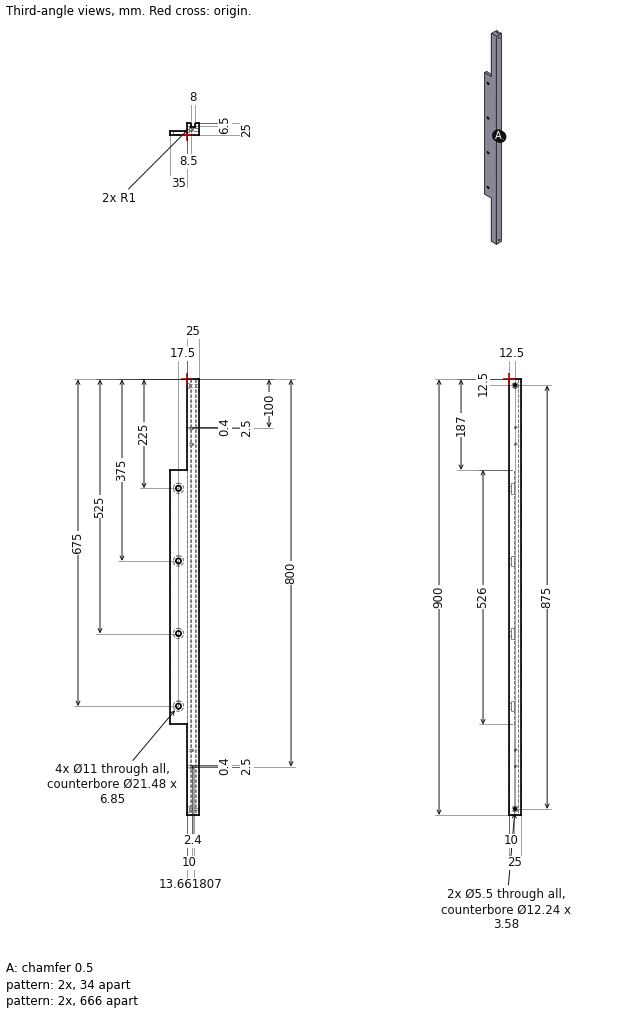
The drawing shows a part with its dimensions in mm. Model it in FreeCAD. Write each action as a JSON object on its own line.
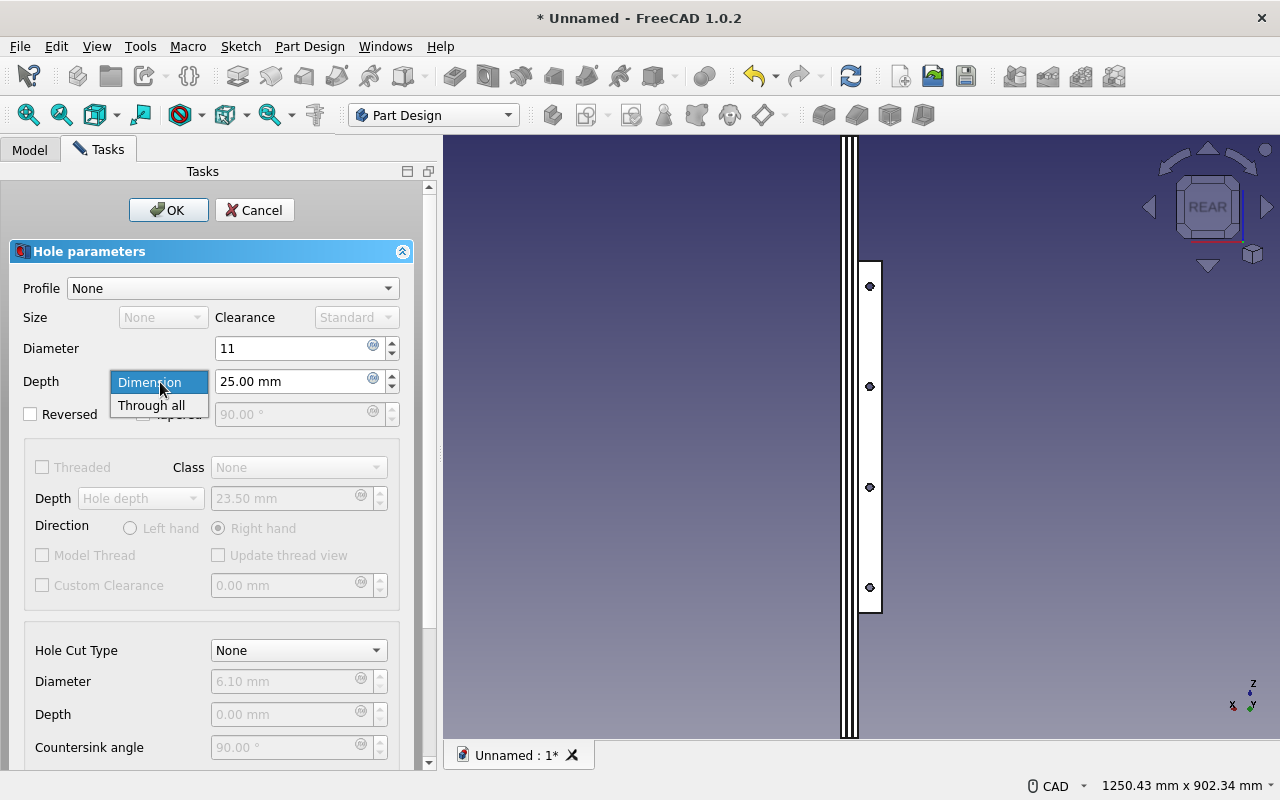
{"action": "left_click", "coordinate": [158, 406]}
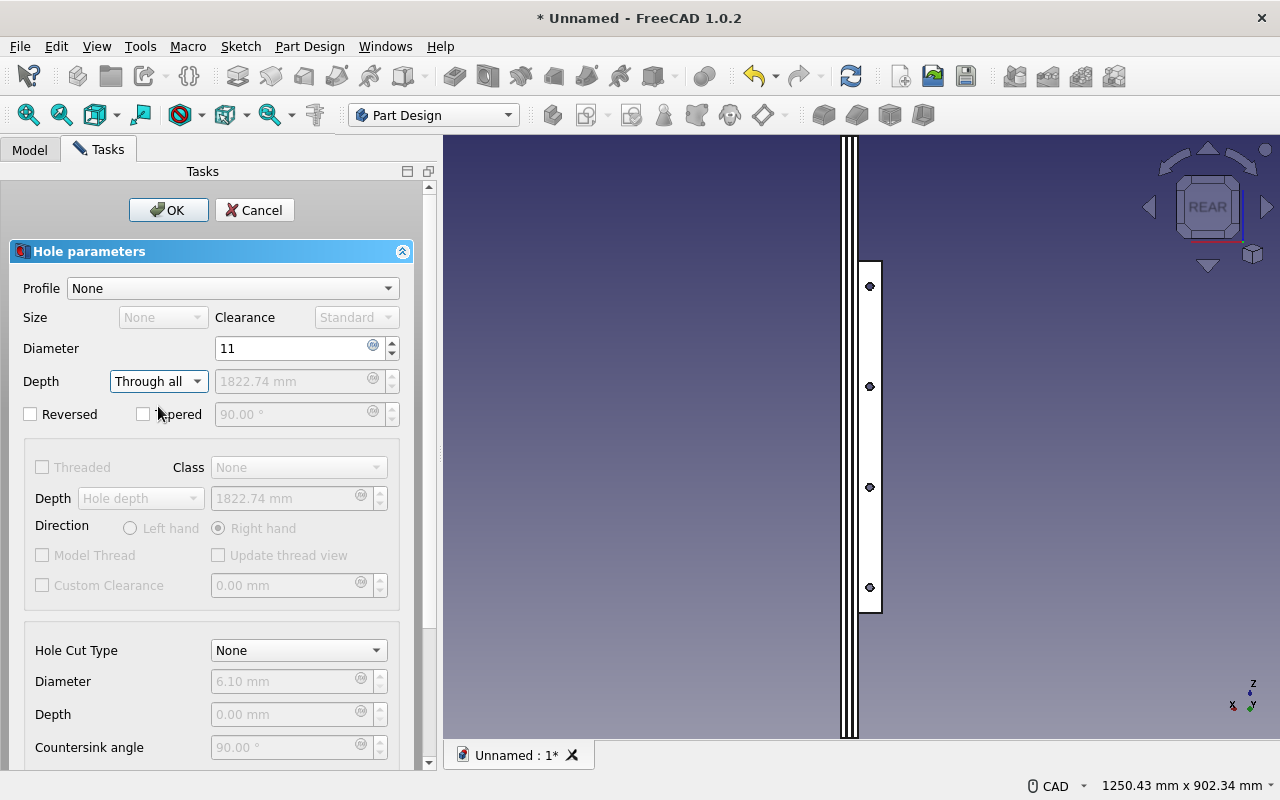
{"action": "left_click", "coordinate": [300, 650]}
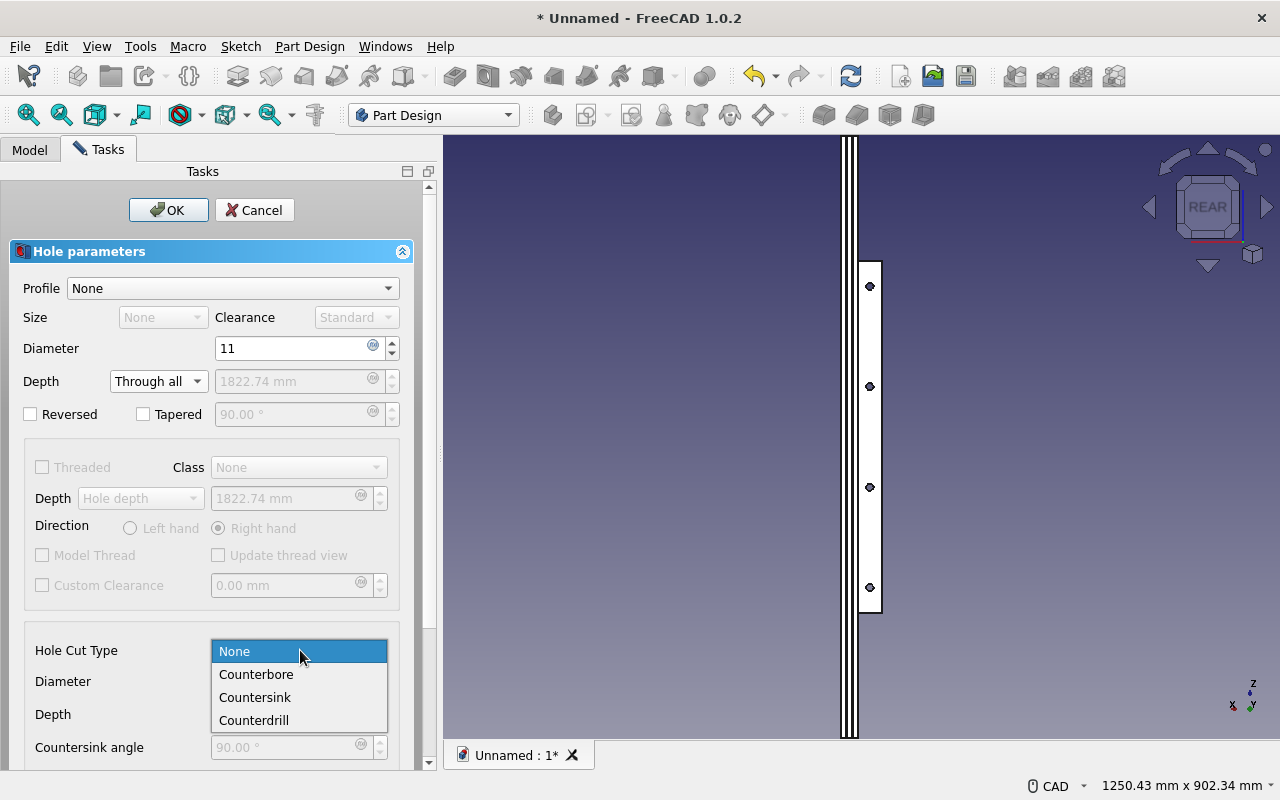
{"action": "left_click", "coordinate": [298, 674]}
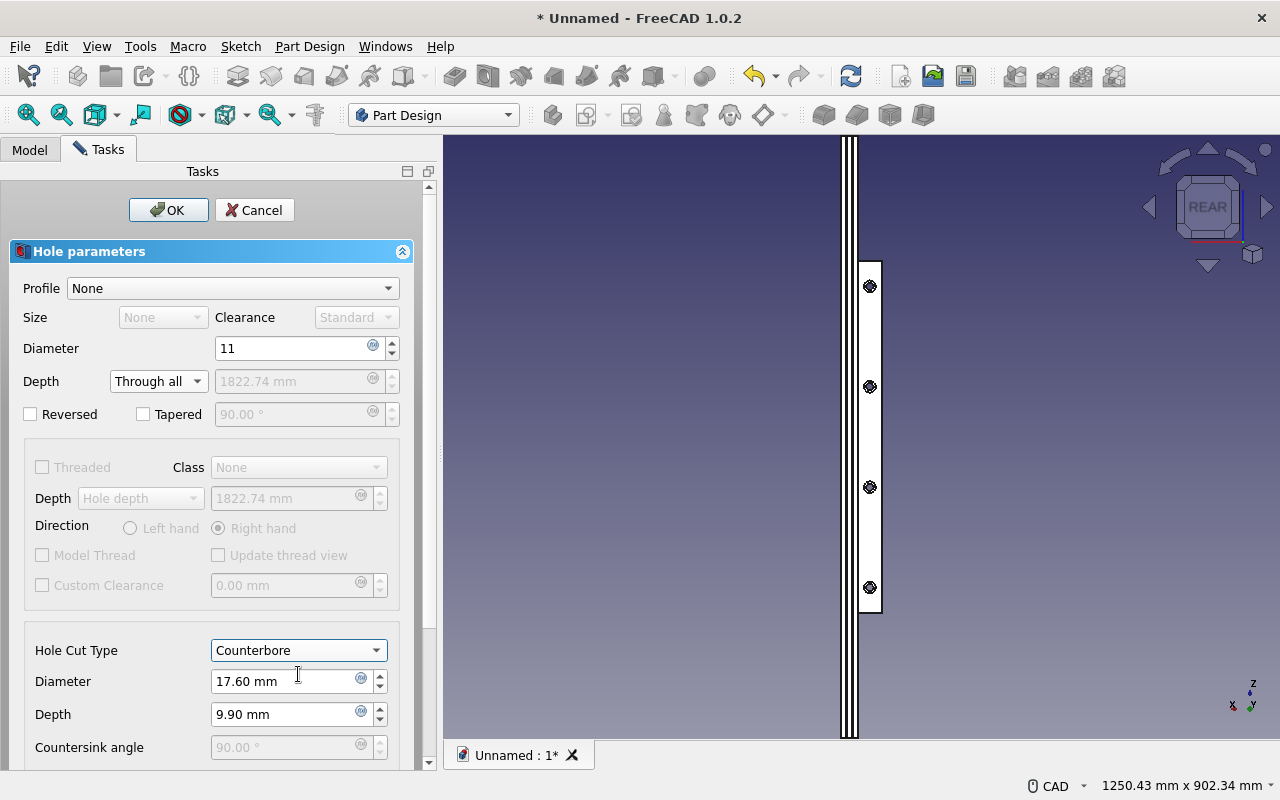
{"action": "triple_click", "coordinate": [292, 682]}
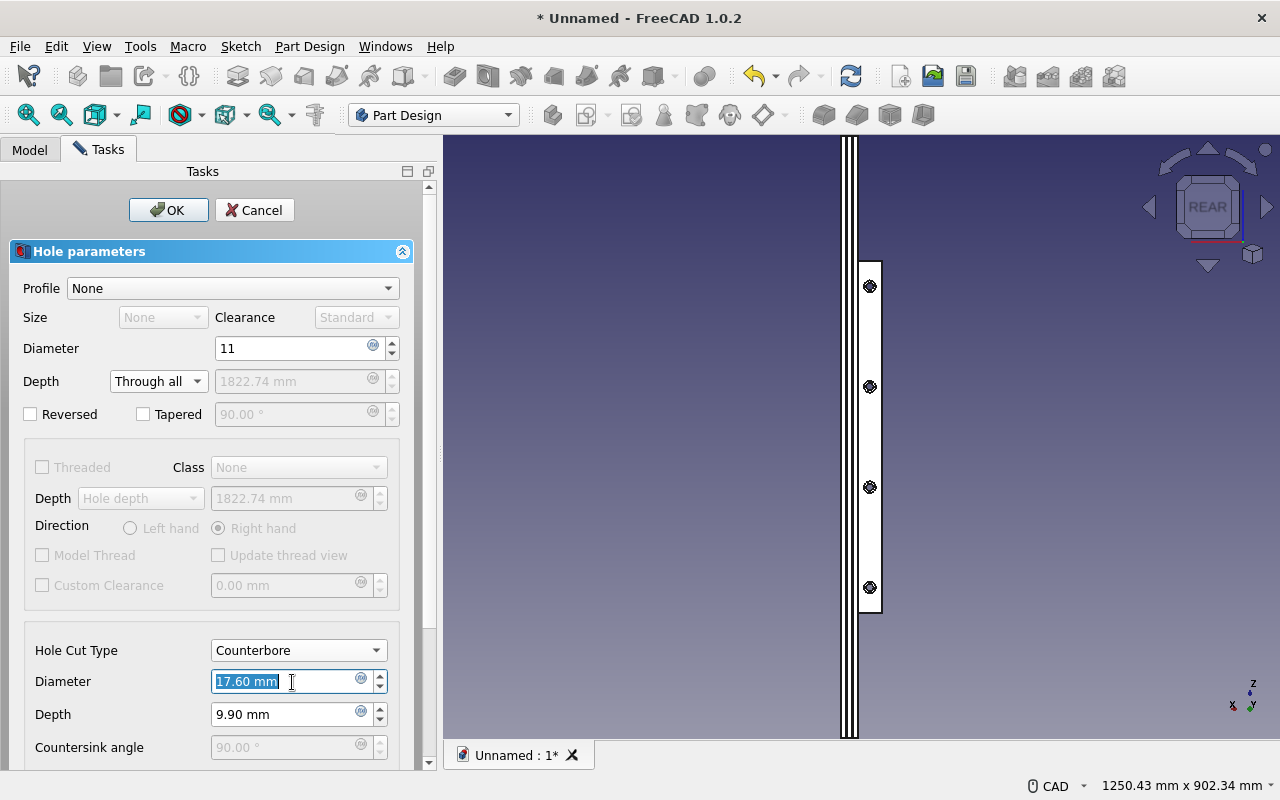
{"action": "type", "text": "21.48"}
{"action": "key", "text": "Tab"}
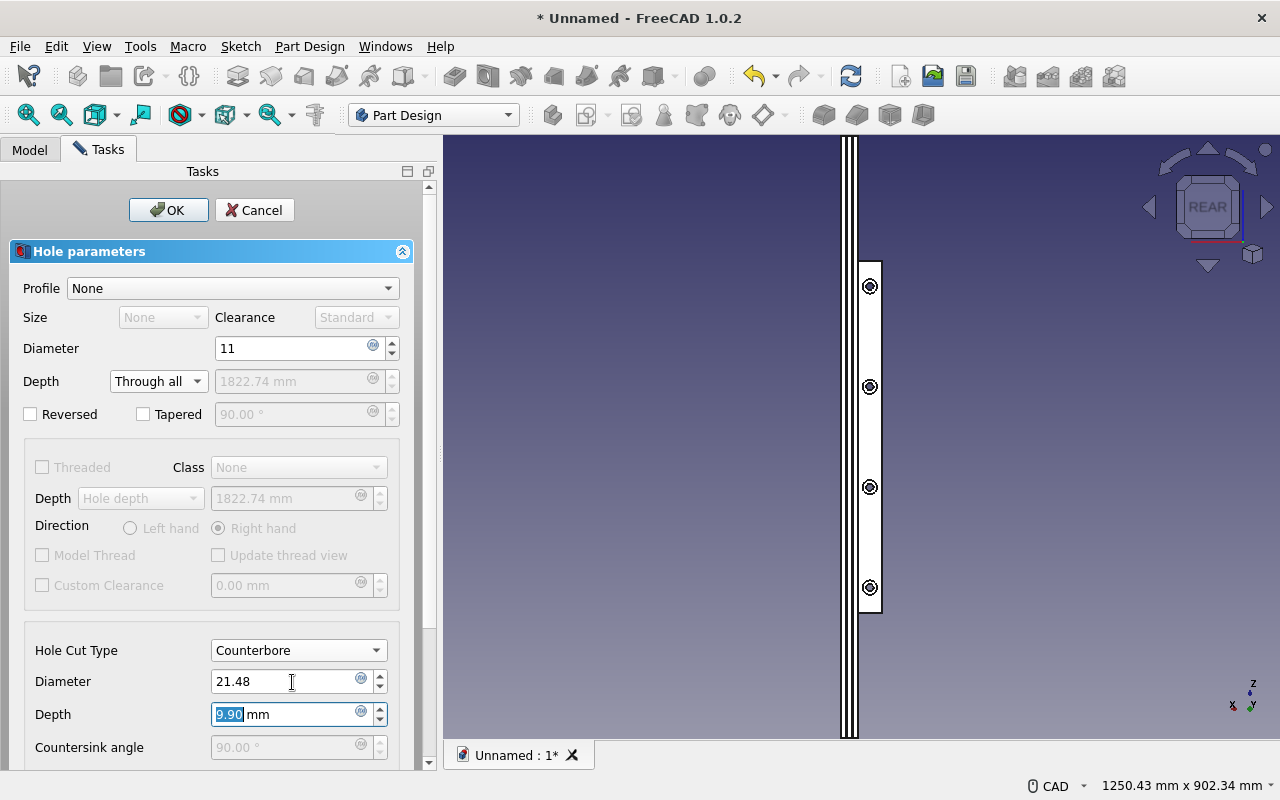
{"action": "type", "text": "6.85"}
{"action": "key", "text": "Tab"}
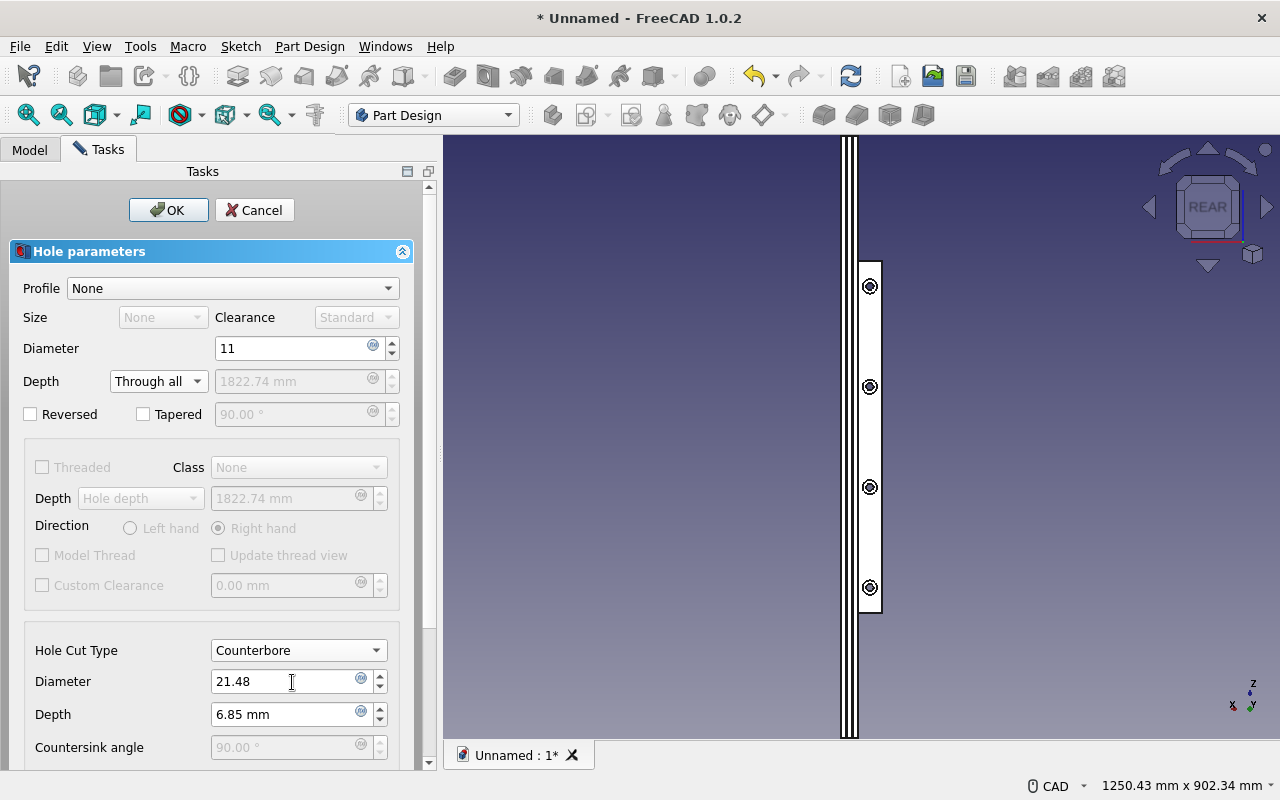
{"action": "left_click", "coordinate": [169, 210]}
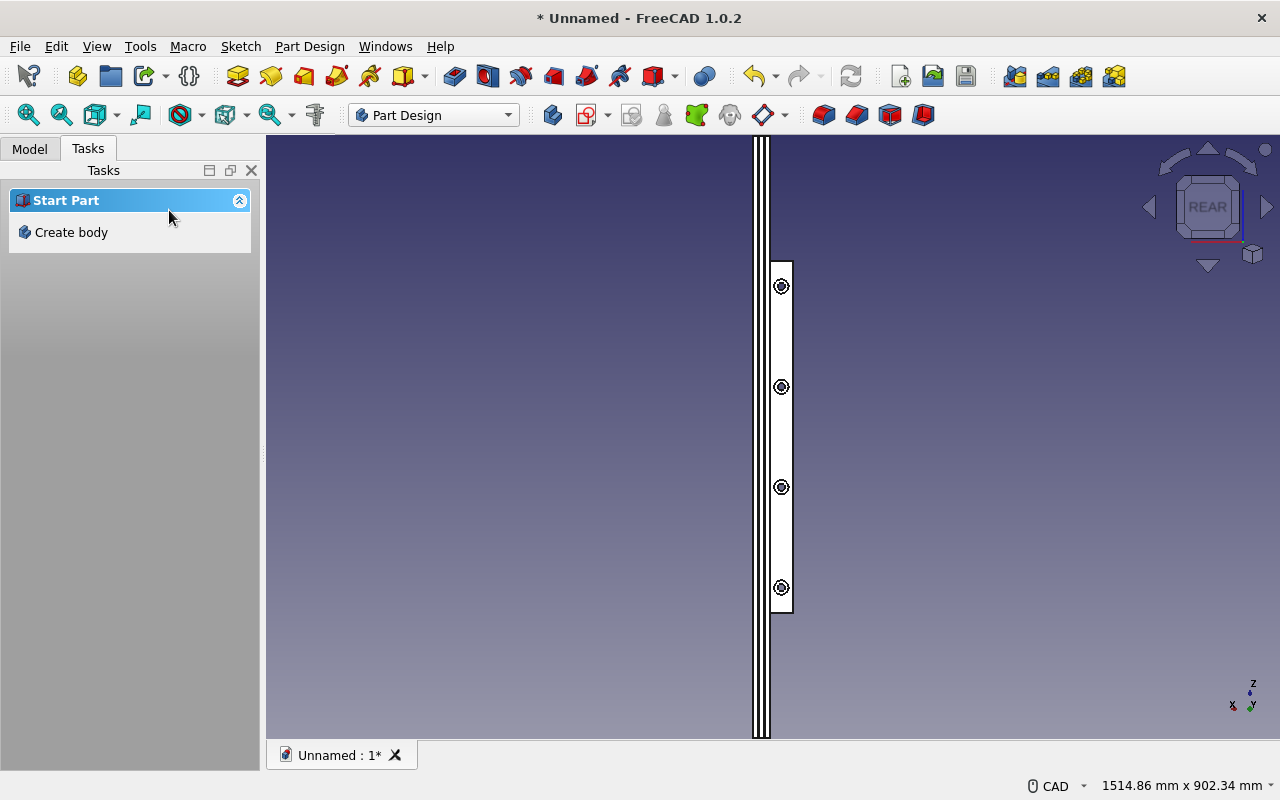
{"action": "key", "text": "6"}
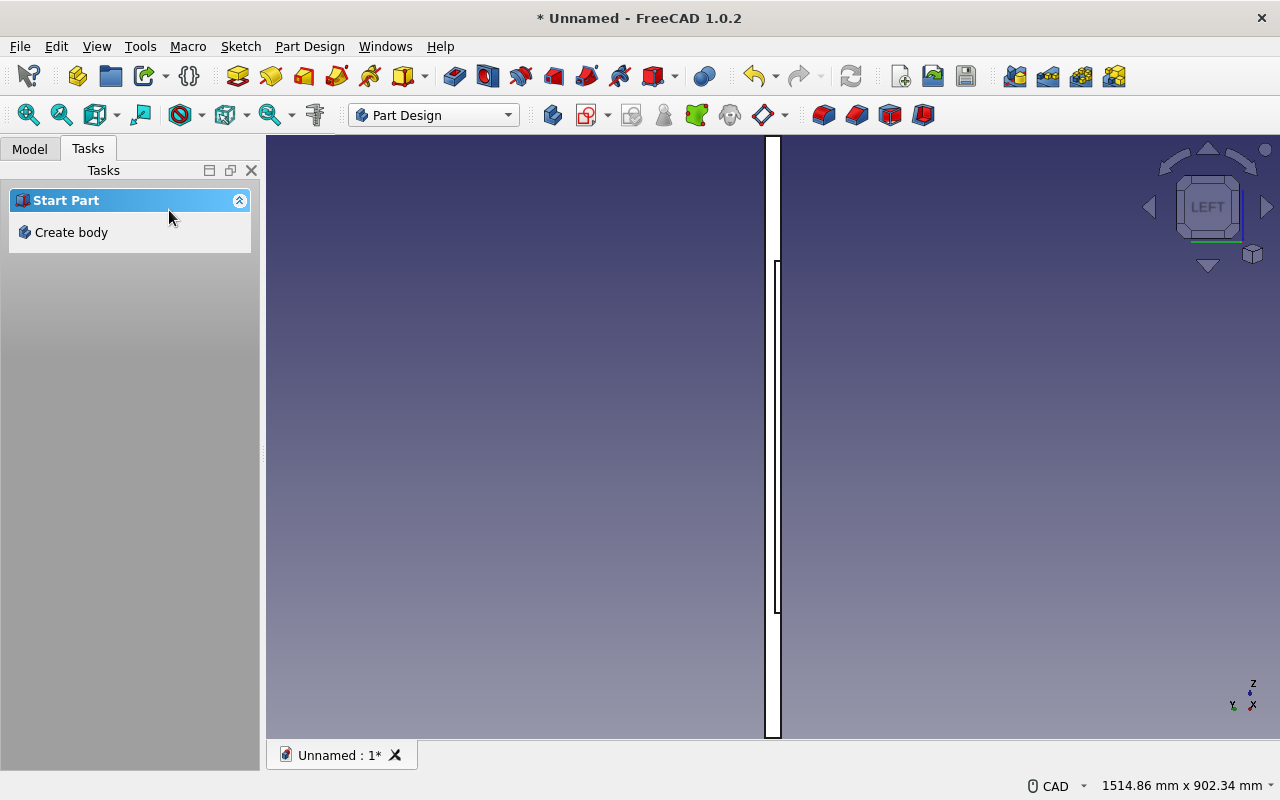
{"action": "left_click", "coordinate": [773, 694]}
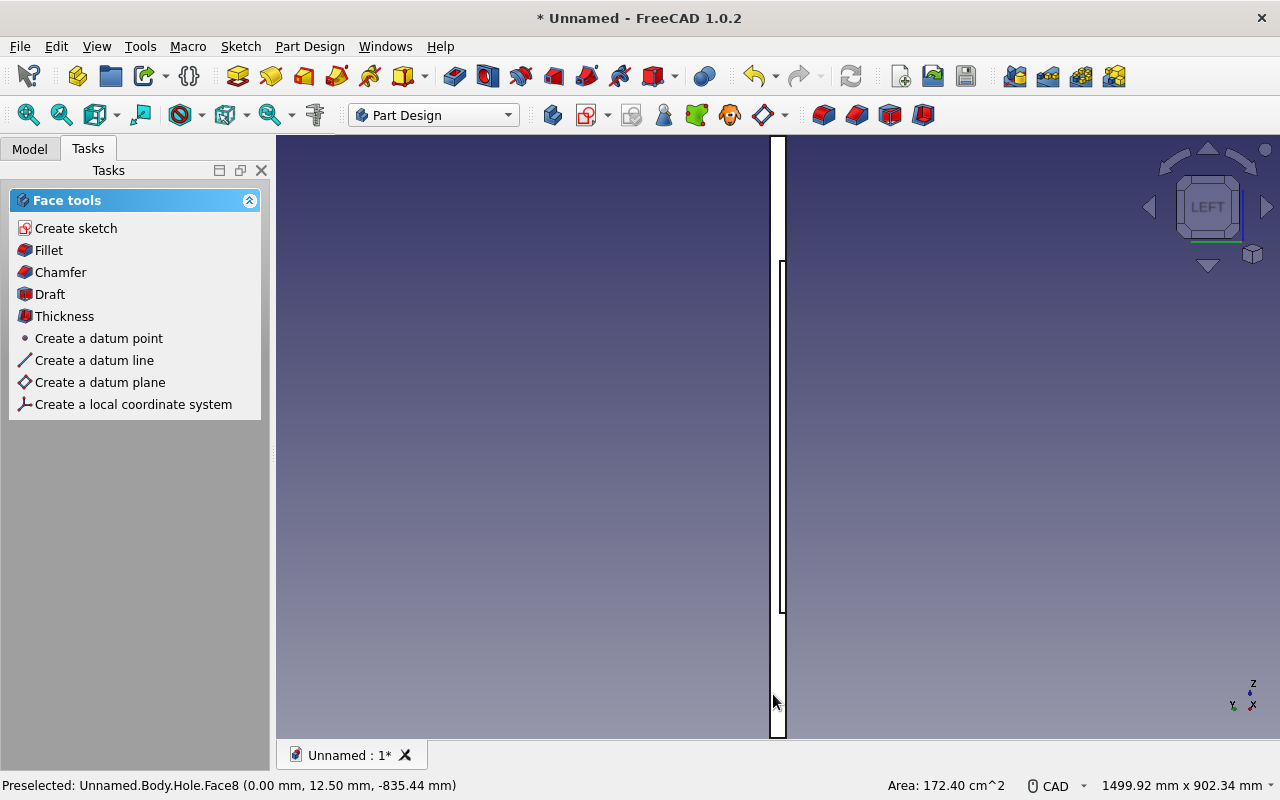
{"action": "left_click", "coordinate": [586, 116]}